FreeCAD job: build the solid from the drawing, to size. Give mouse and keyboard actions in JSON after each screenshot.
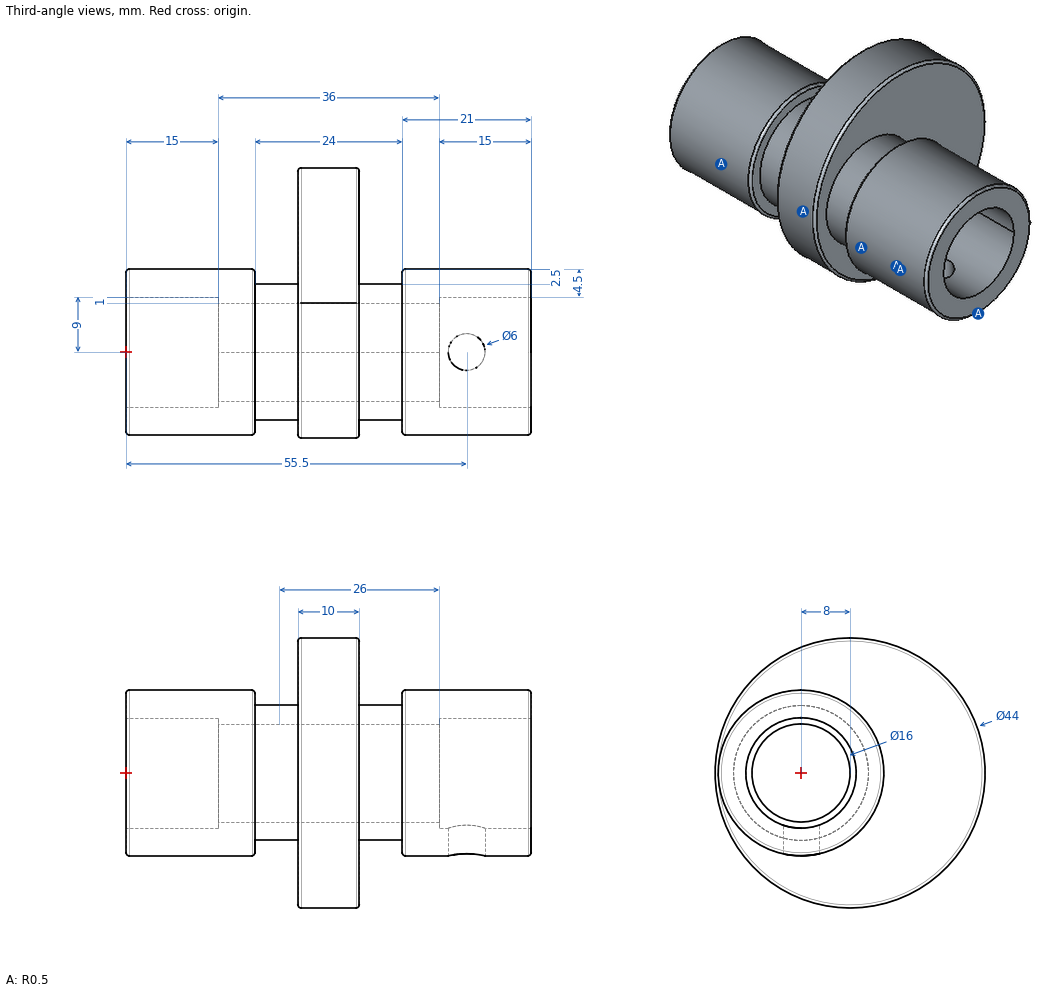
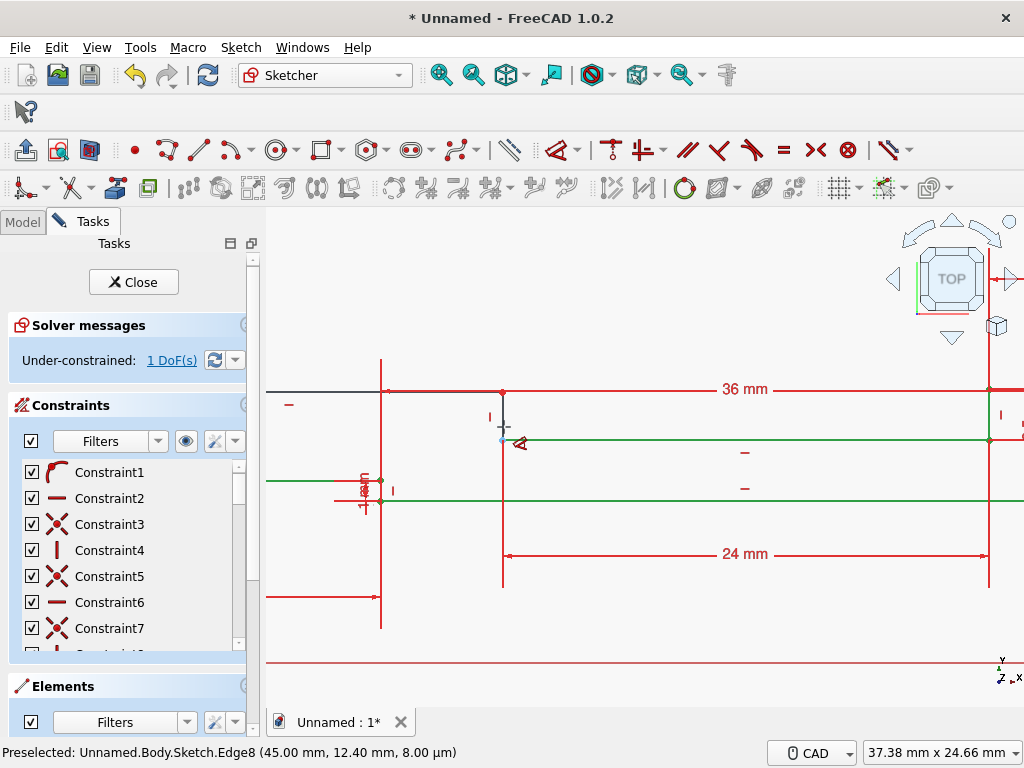
{"action": "left_click", "coordinate": [503, 426]}
{"action": "left_click", "coordinate": [469, 416]}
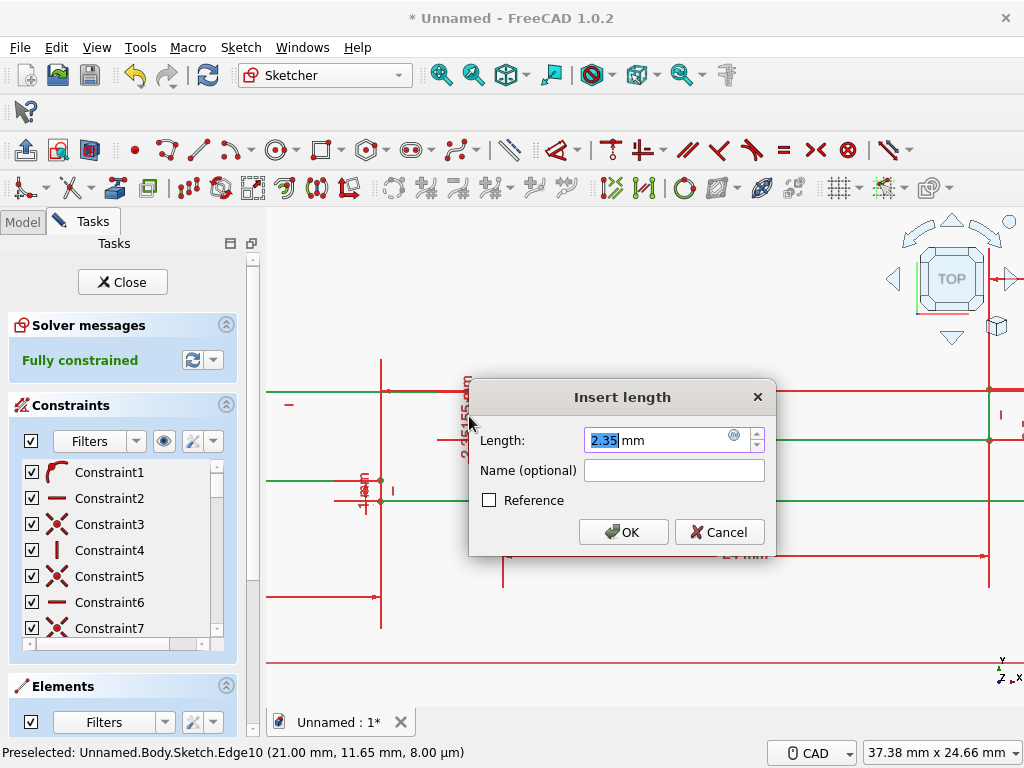
{"action": "type", "text": "2.5"}
{"action": "key", "text": "Return"}
{"action": "key", "text": "Escape"}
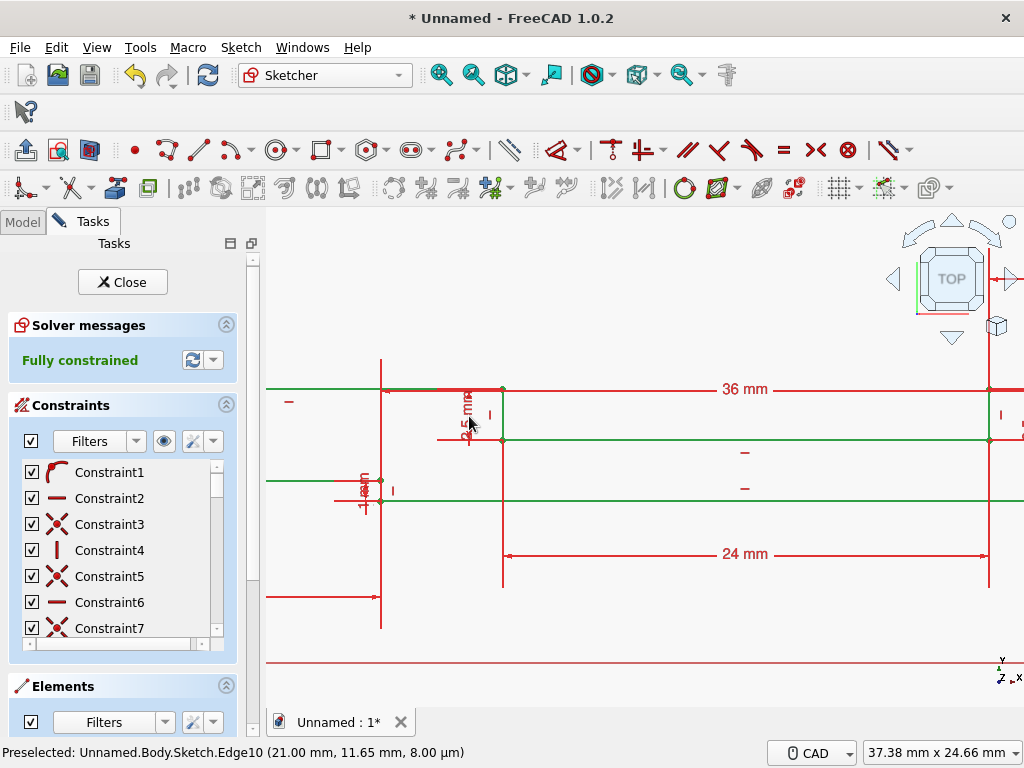
{"action": "left_click", "coordinate": [123, 282]}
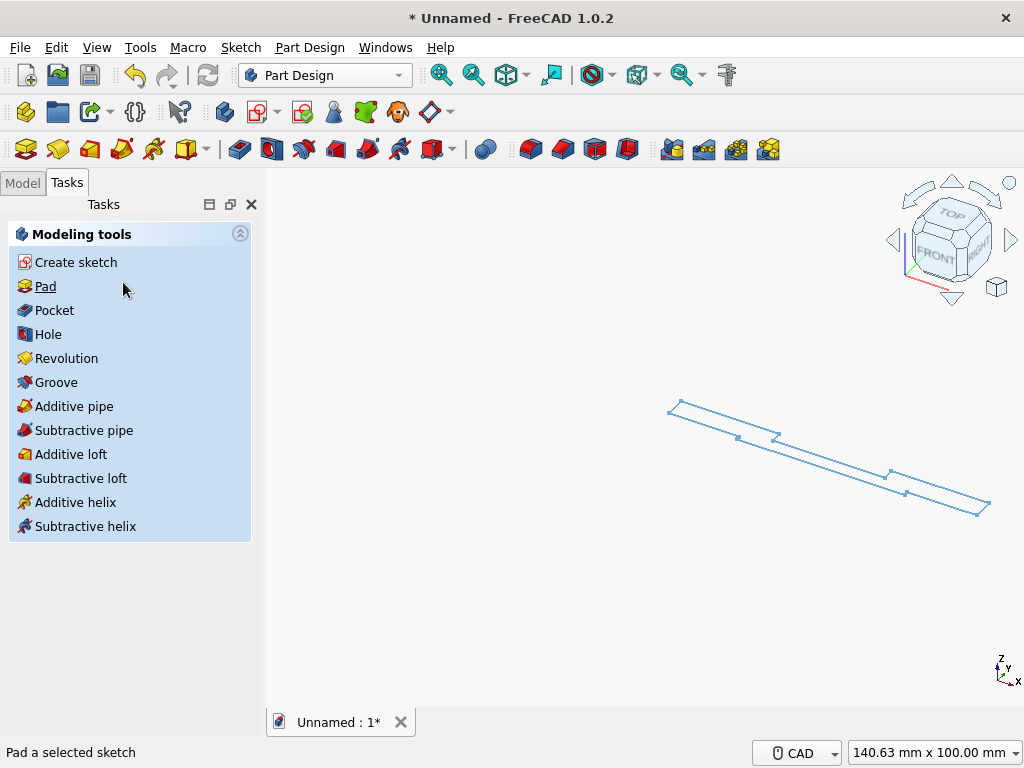
{"action": "left_click", "coordinate": [58, 150]}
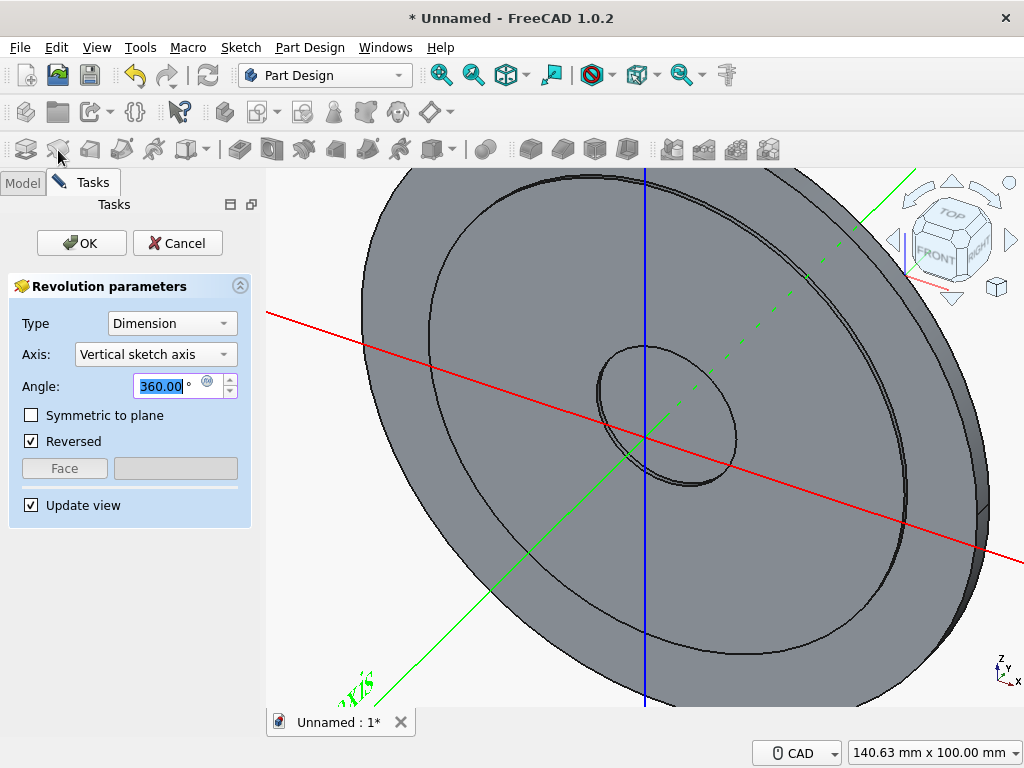
{"action": "left_click", "coordinate": [156, 354]}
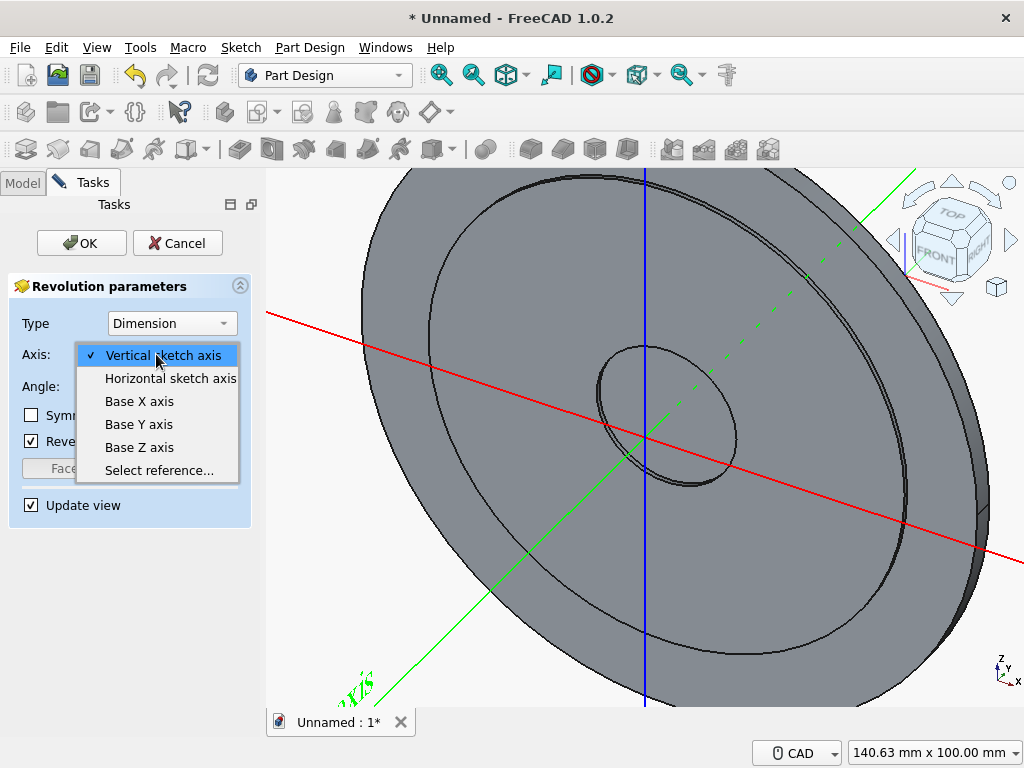
{"action": "left_click", "coordinate": [156, 378]}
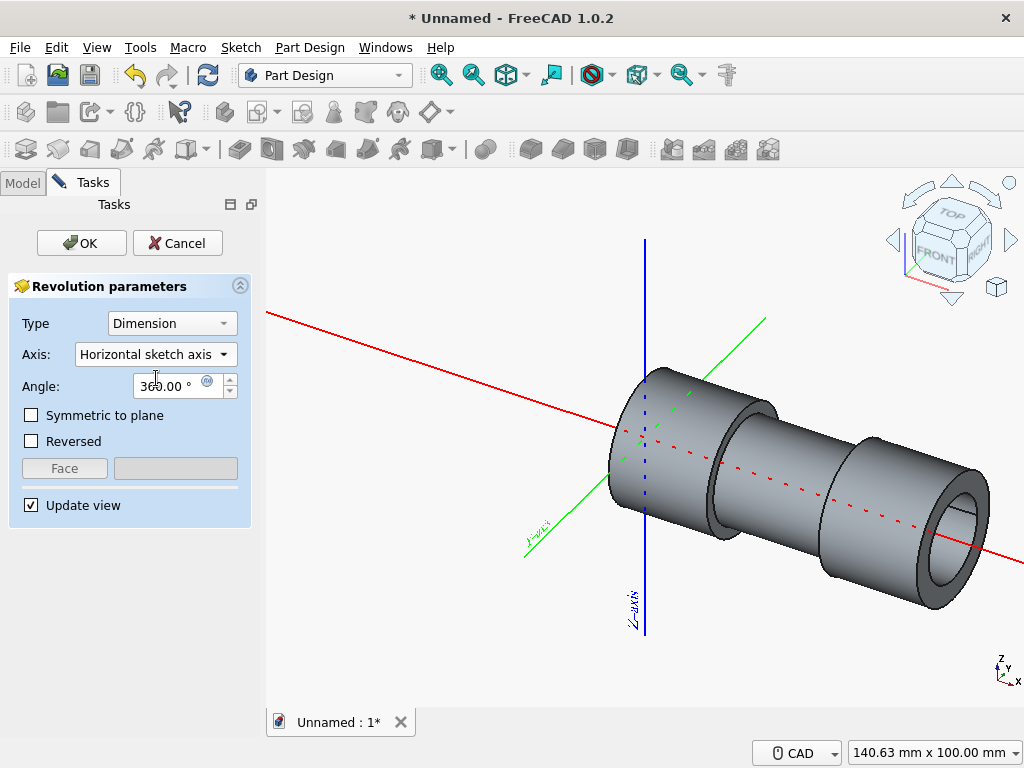
{"action": "left_click", "coordinate": [82, 243]}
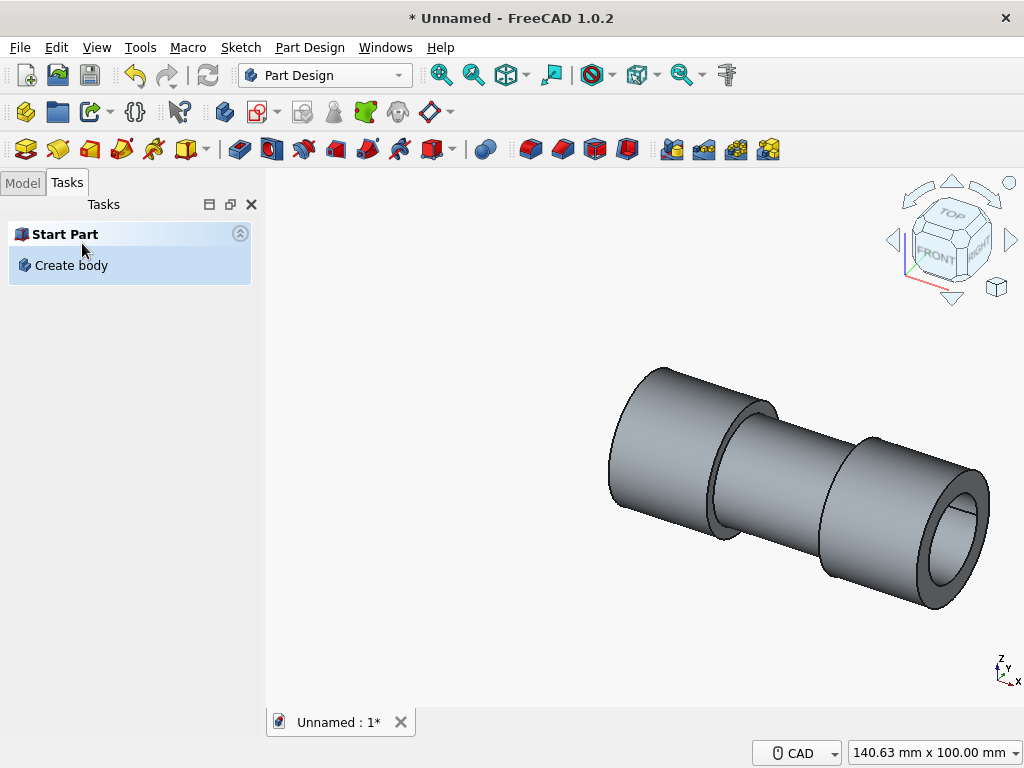
{"action": "left_click", "coordinate": [23, 182]}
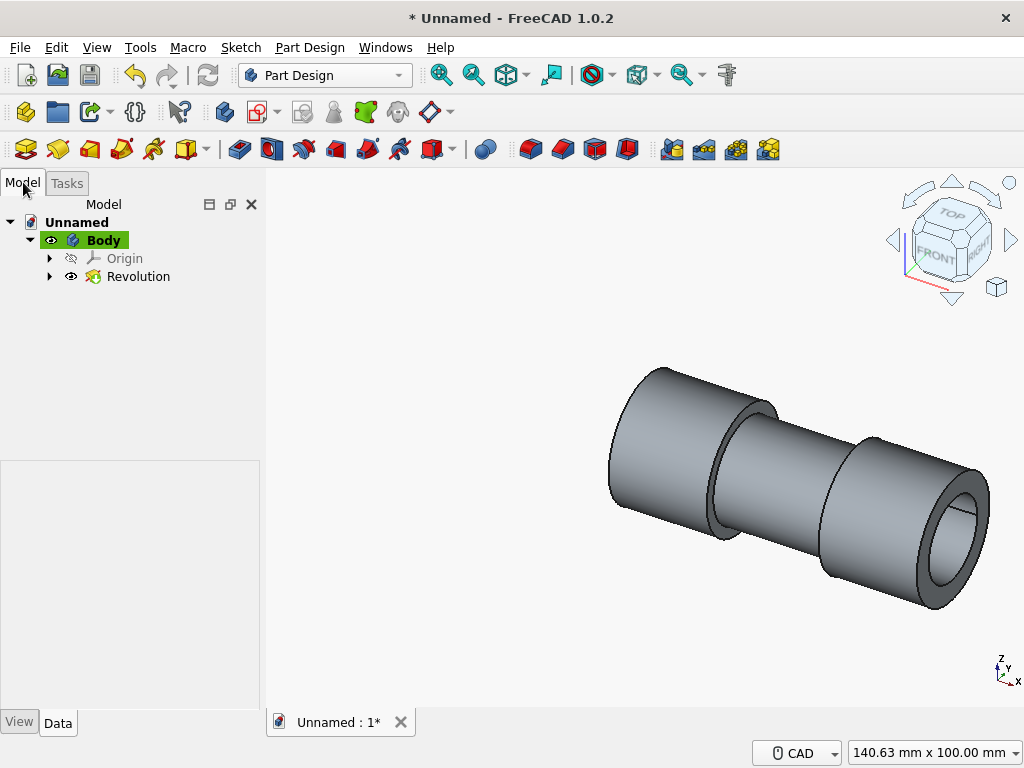
{"action": "left_click", "coordinate": [50, 258]}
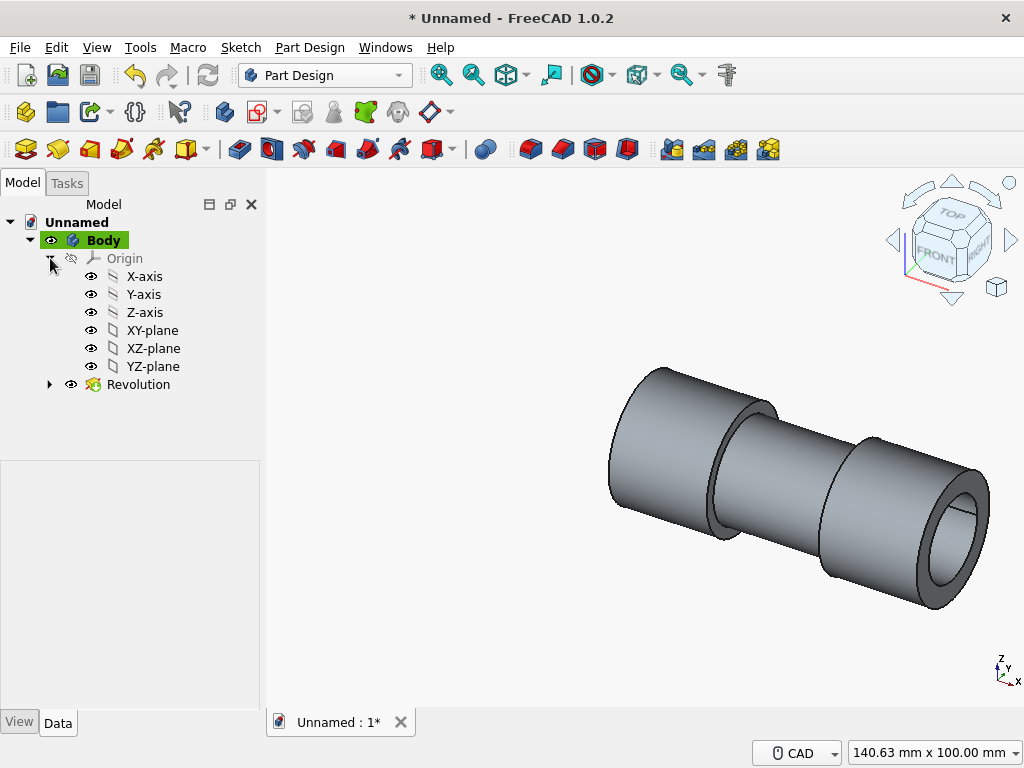
{"action": "left_click", "coordinate": [136, 366]}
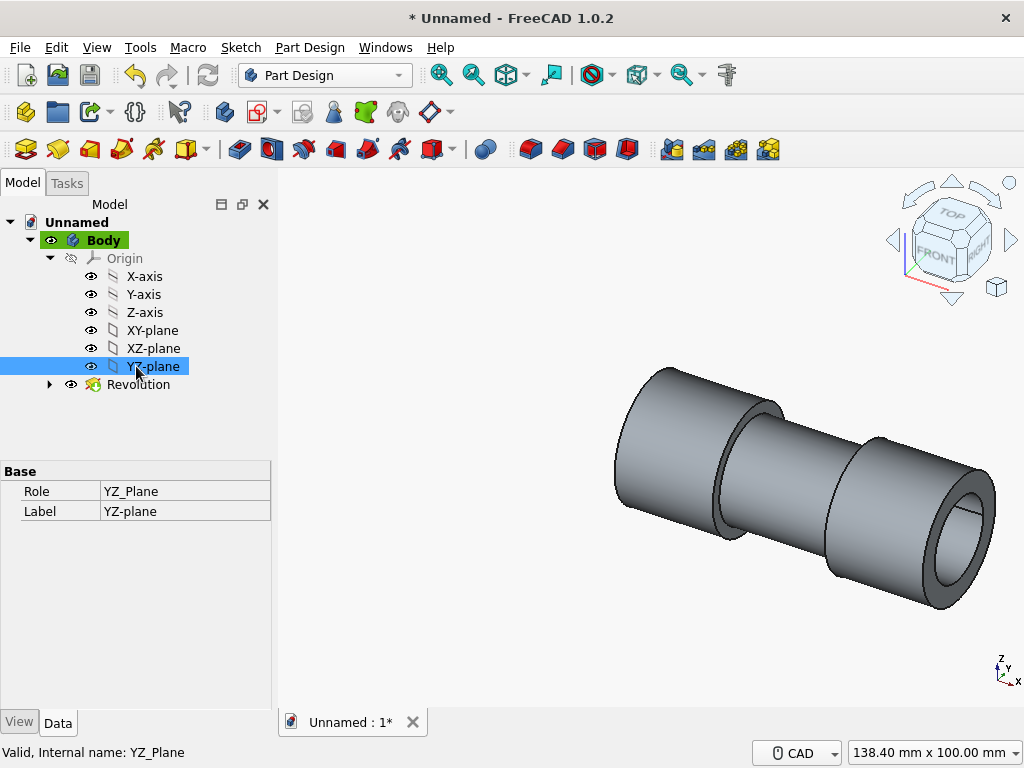
{"action": "left_click", "coordinate": [430, 112]}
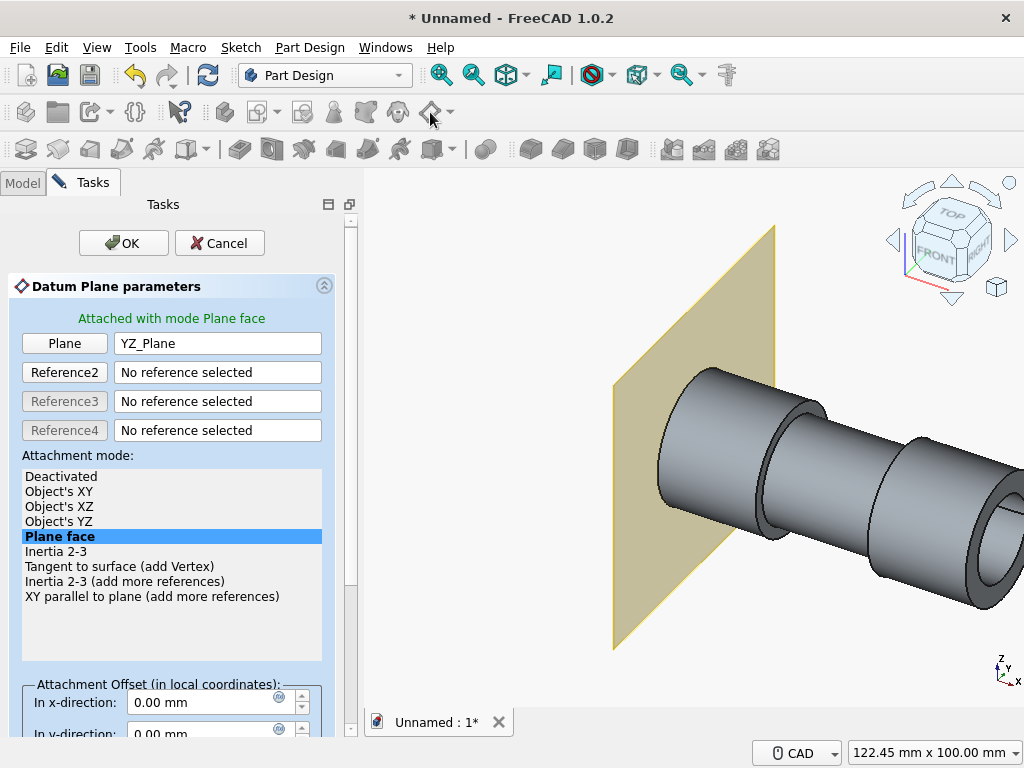
{"action": "scroll", "coordinate": [351, 475], "scroll_direction": "down", "scroll_amount": 2}